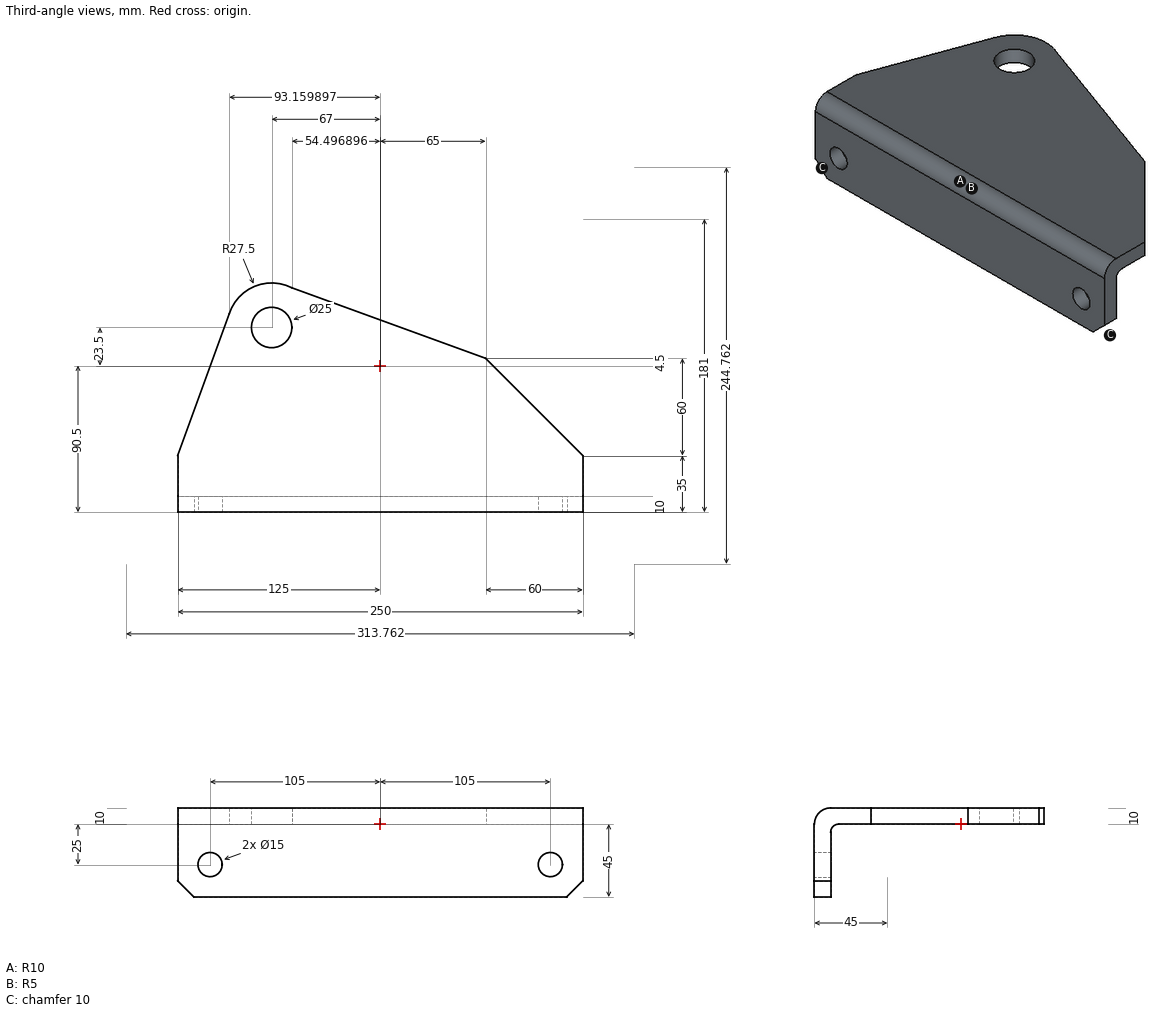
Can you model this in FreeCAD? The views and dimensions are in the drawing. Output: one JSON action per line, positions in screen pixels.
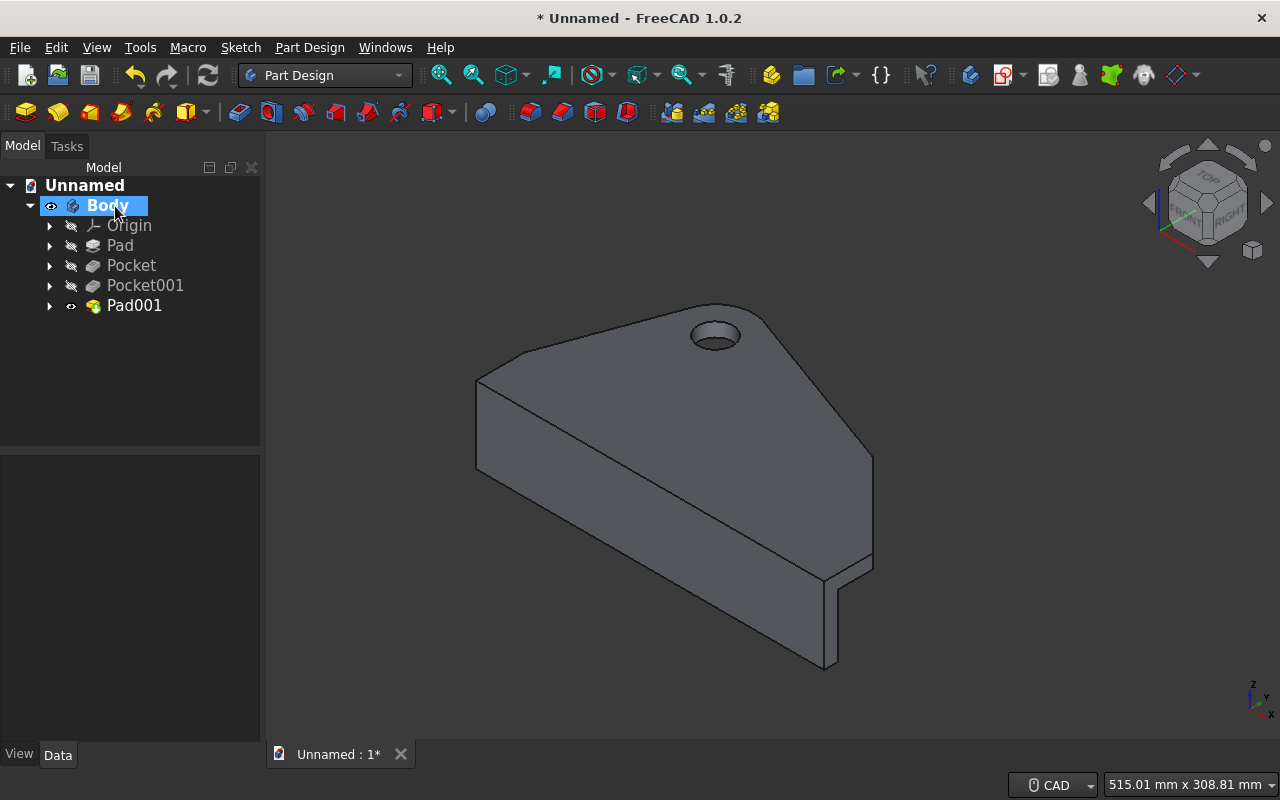
{"action": "left_click", "coordinate": [650, 480]}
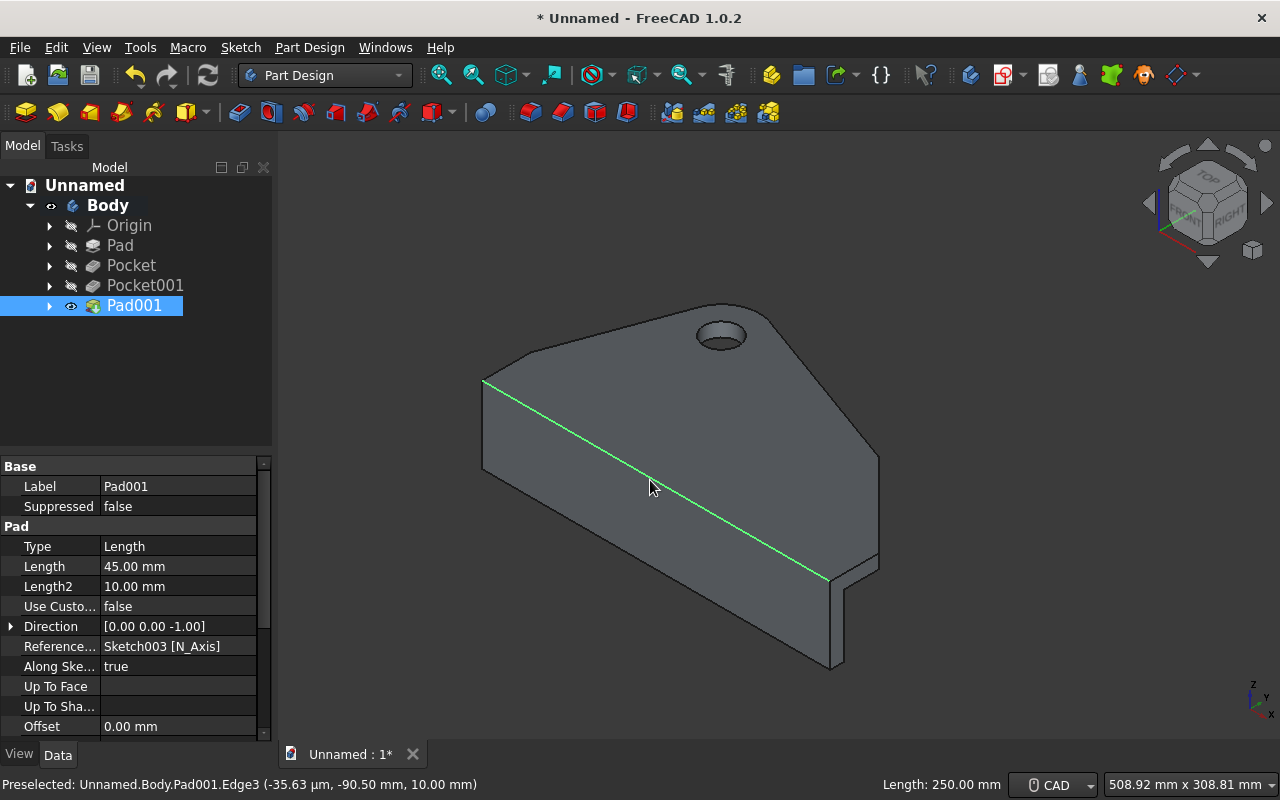
{"action": "left_click", "coordinate": [532, 112]}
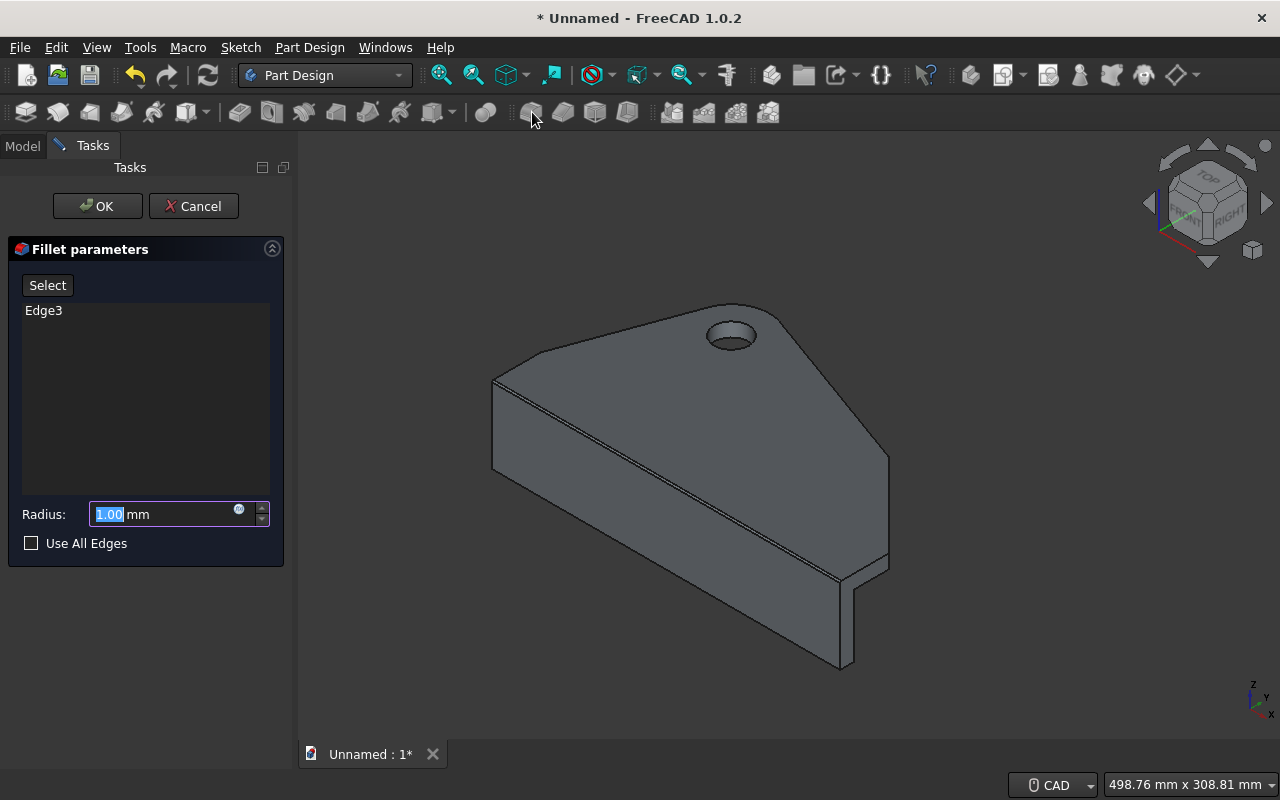
{"action": "type", "text": "10"}
{"action": "key", "text": "Tab"}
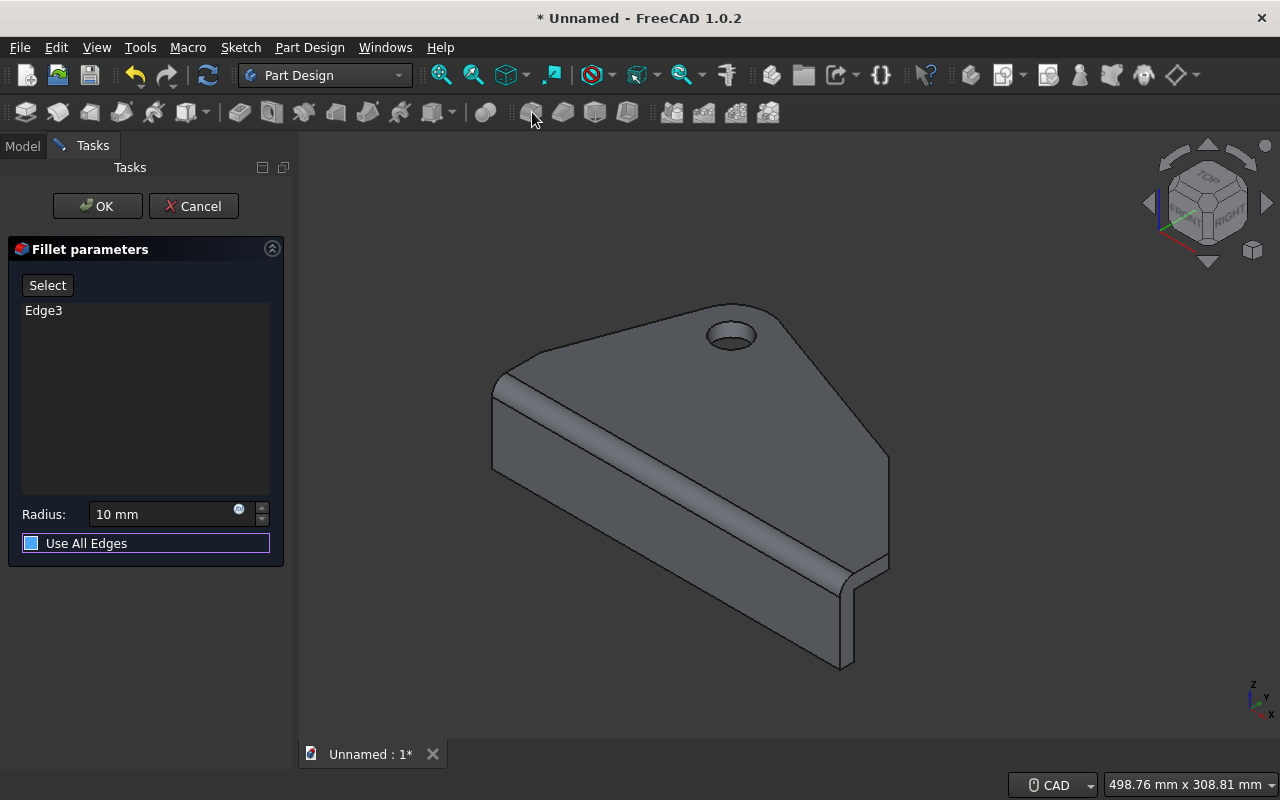
{"action": "left_click", "coordinate": [98, 206]}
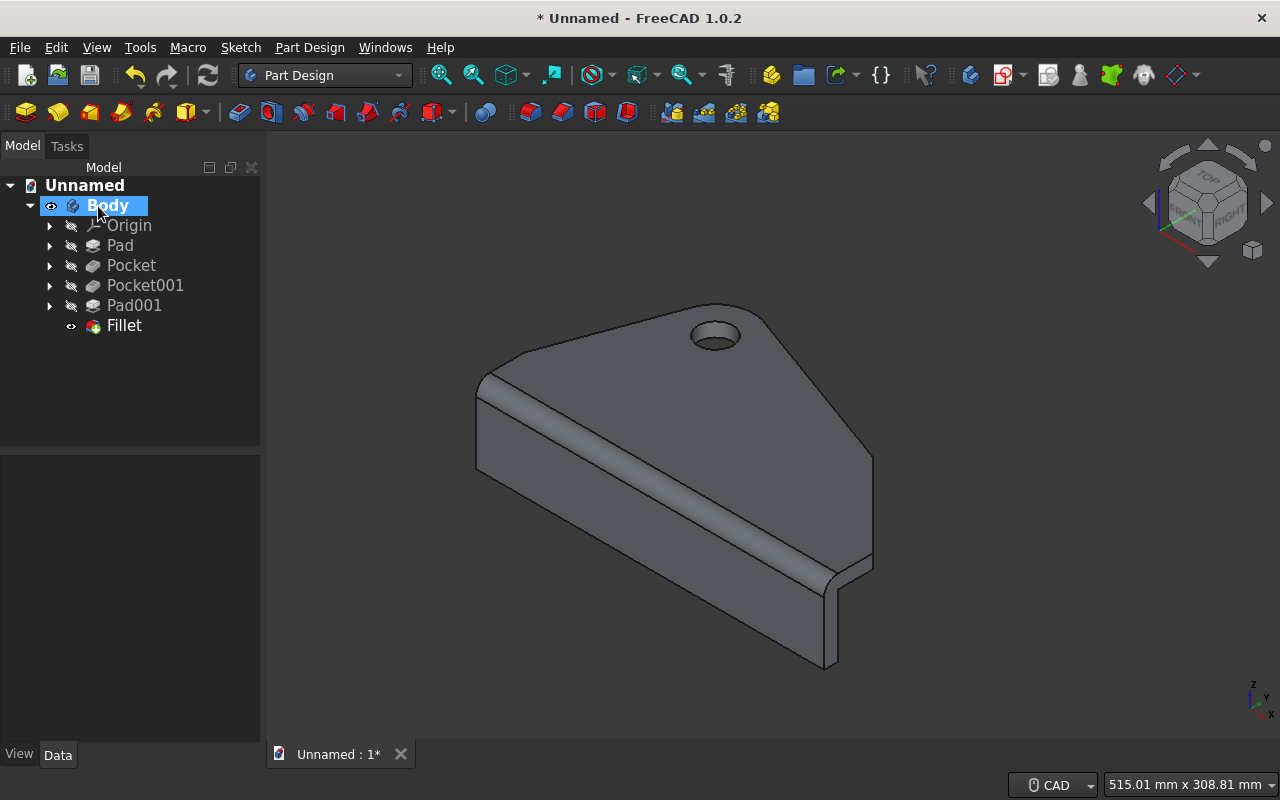
{"action": "key", "text": "2"}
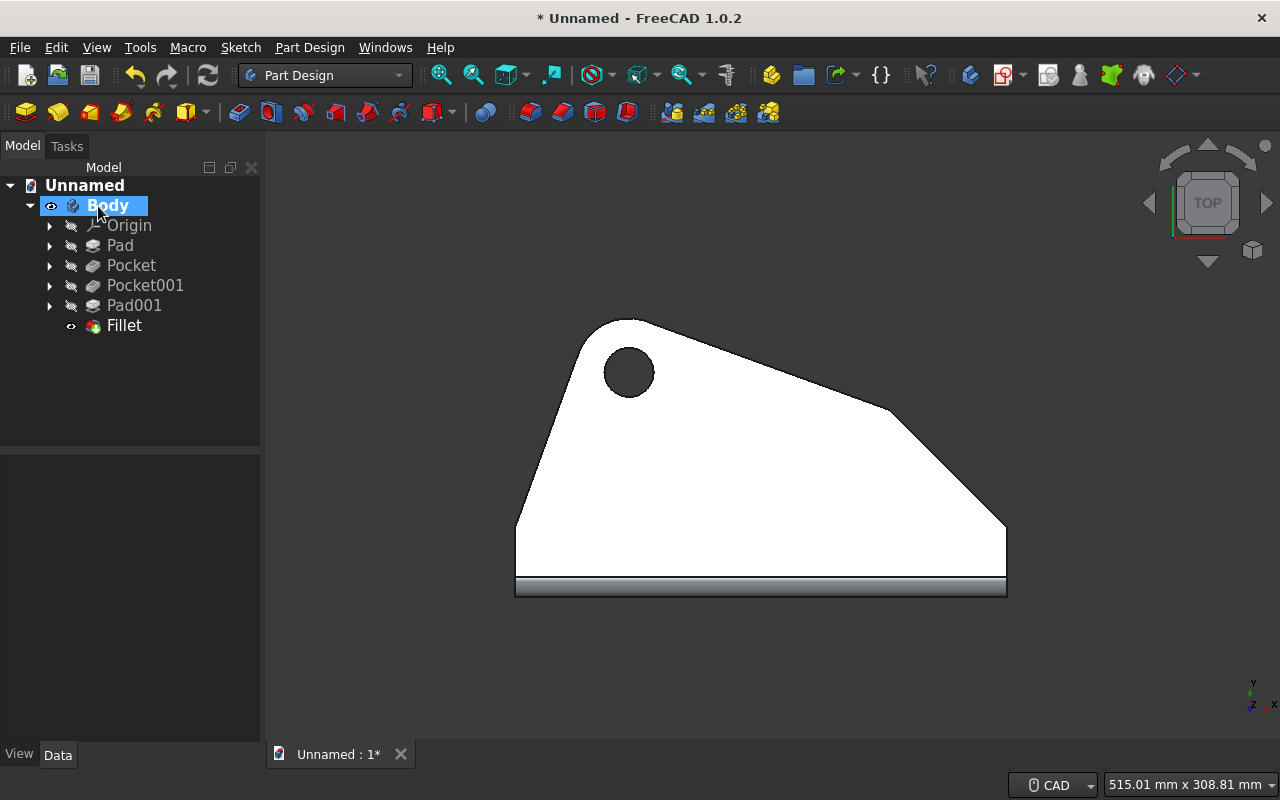
{"action": "key", "text": "0"}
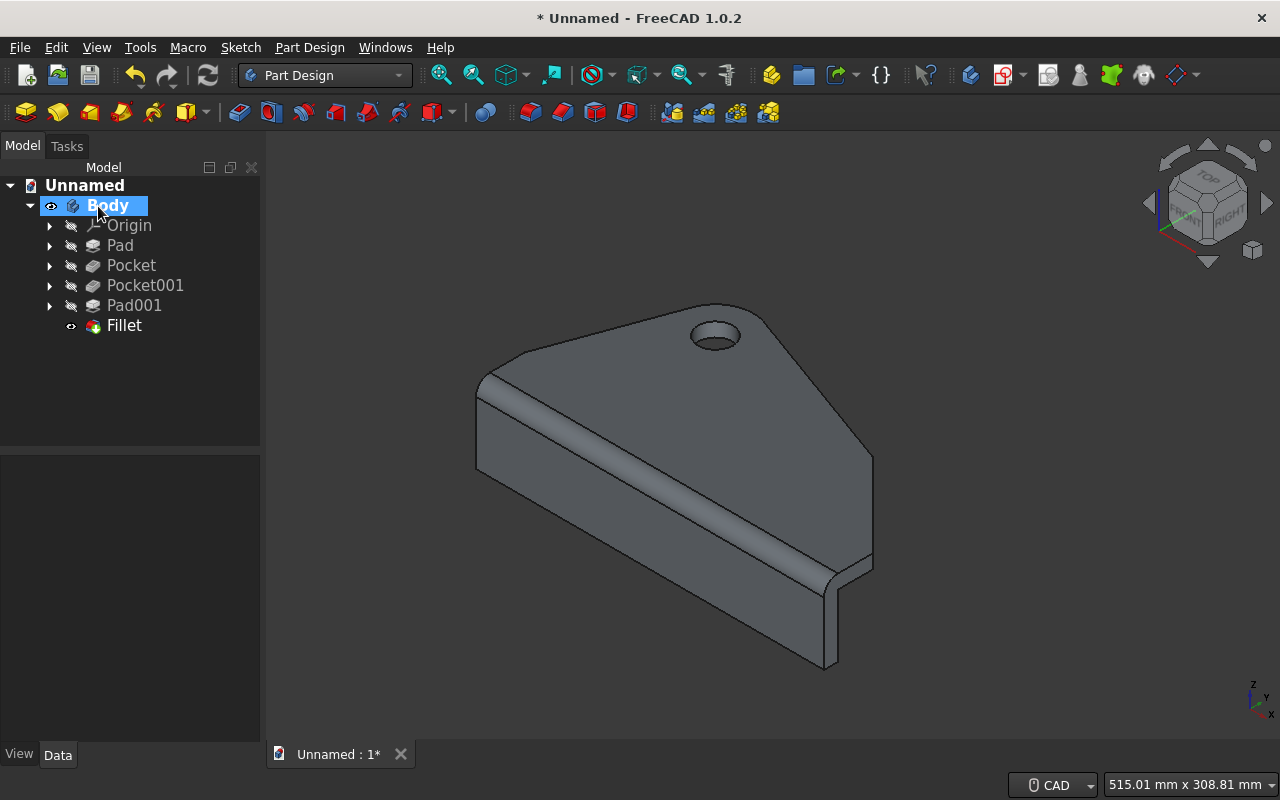
{"action": "key", "text": "1"}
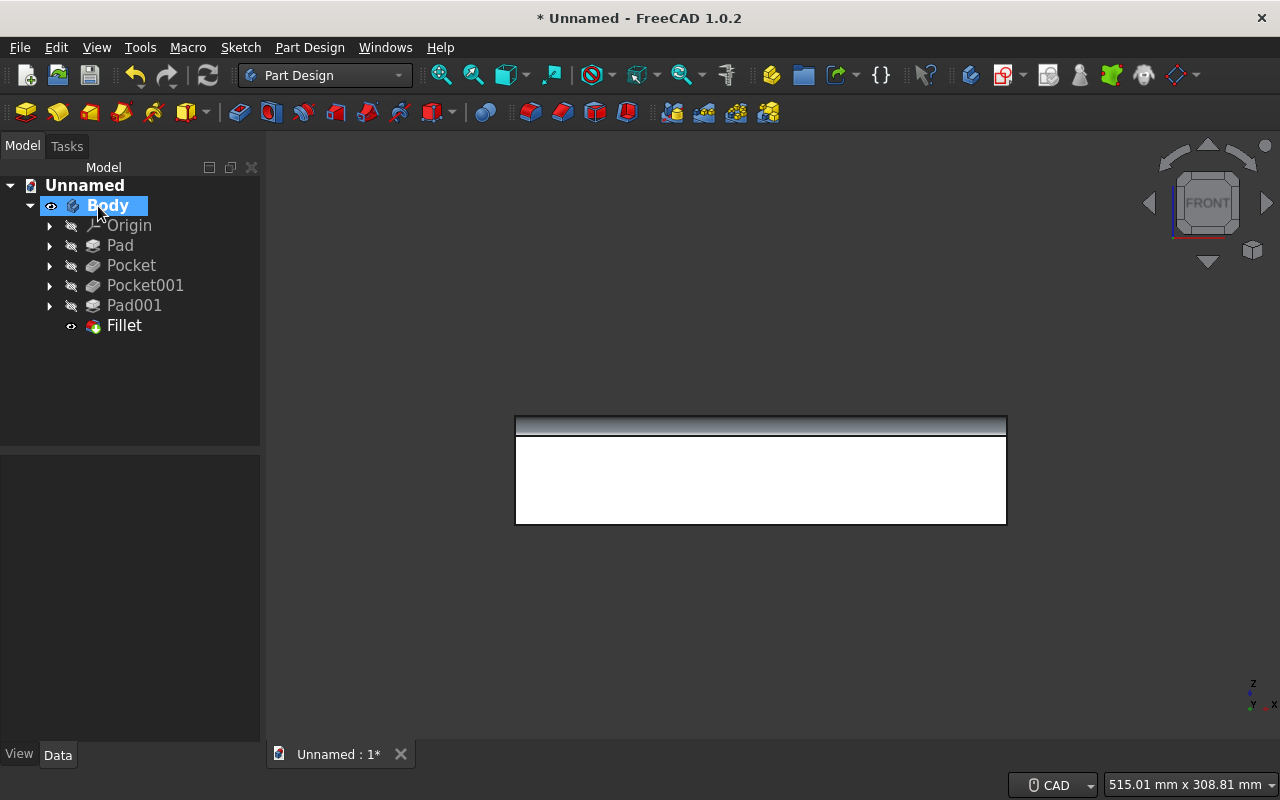
{"action": "key", "text": "3"}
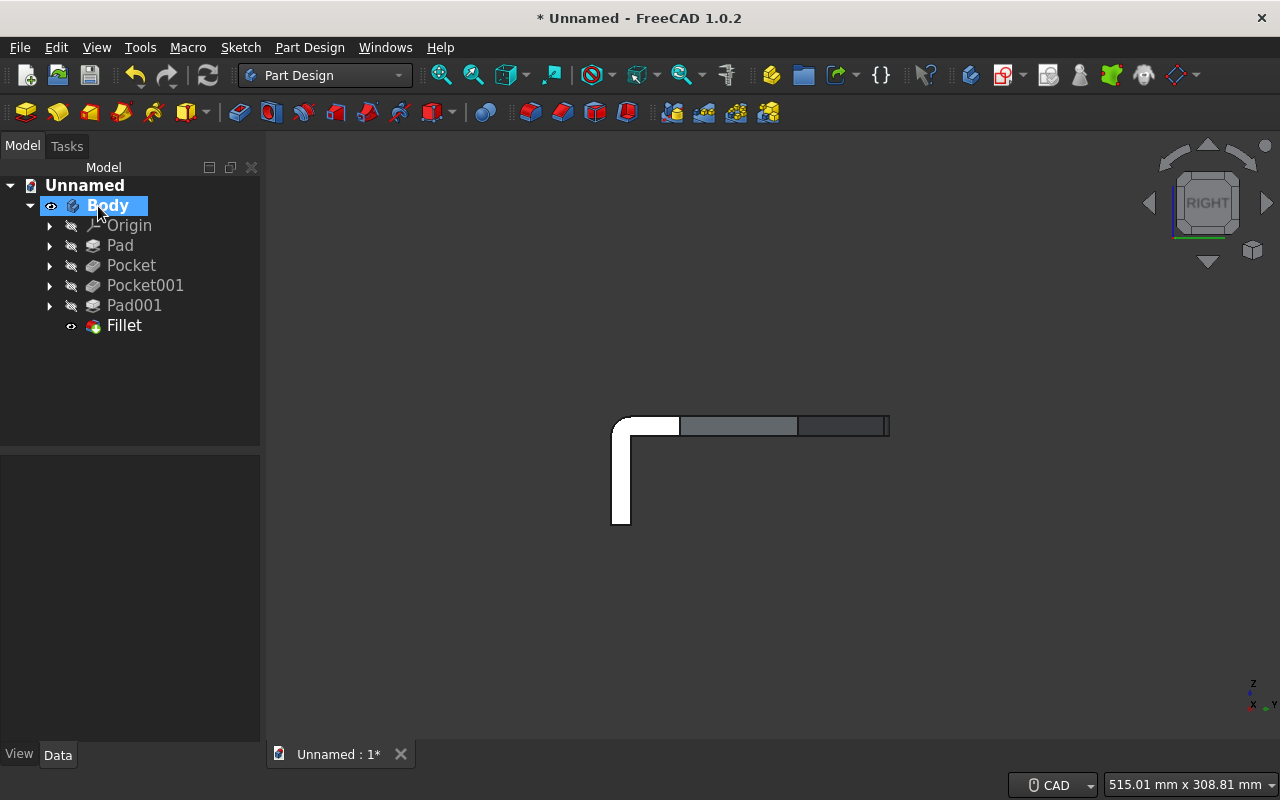
{"action": "key", "text": "v f"}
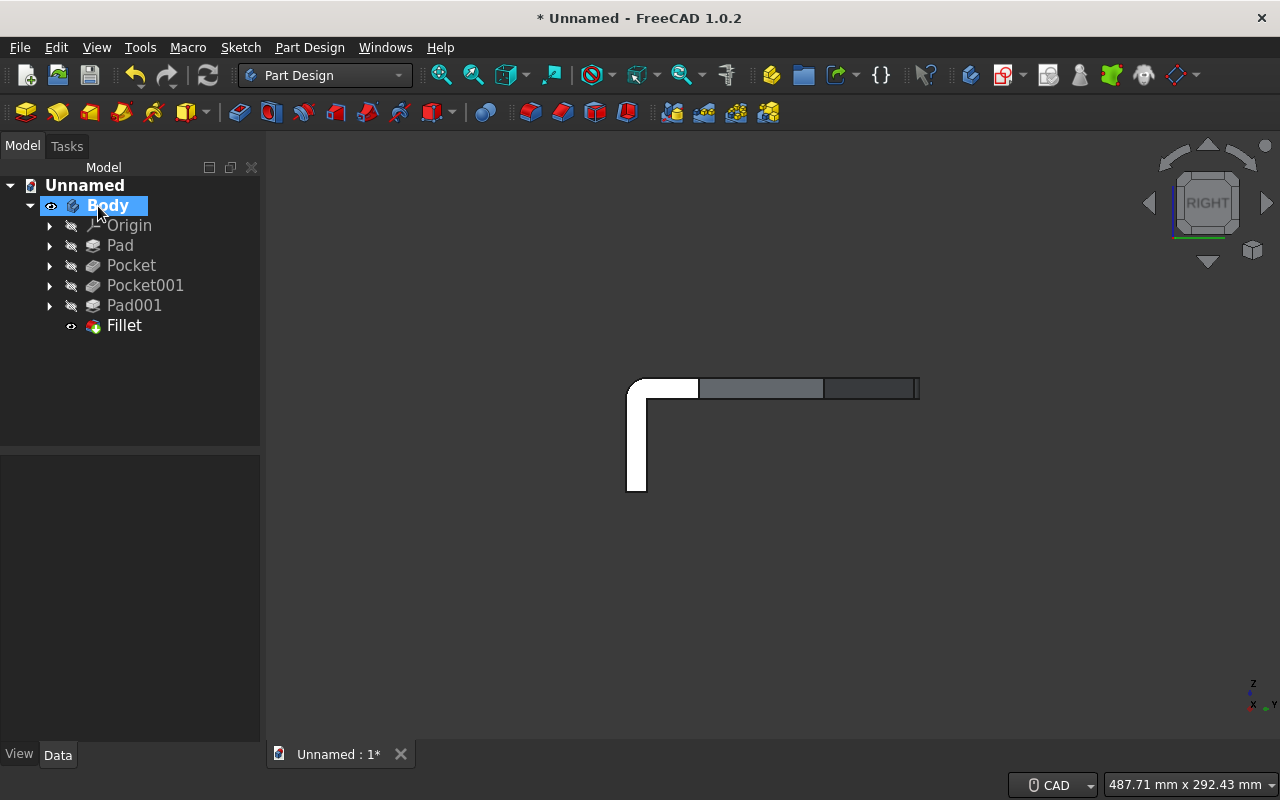
{"action": "key", "text": "5"}